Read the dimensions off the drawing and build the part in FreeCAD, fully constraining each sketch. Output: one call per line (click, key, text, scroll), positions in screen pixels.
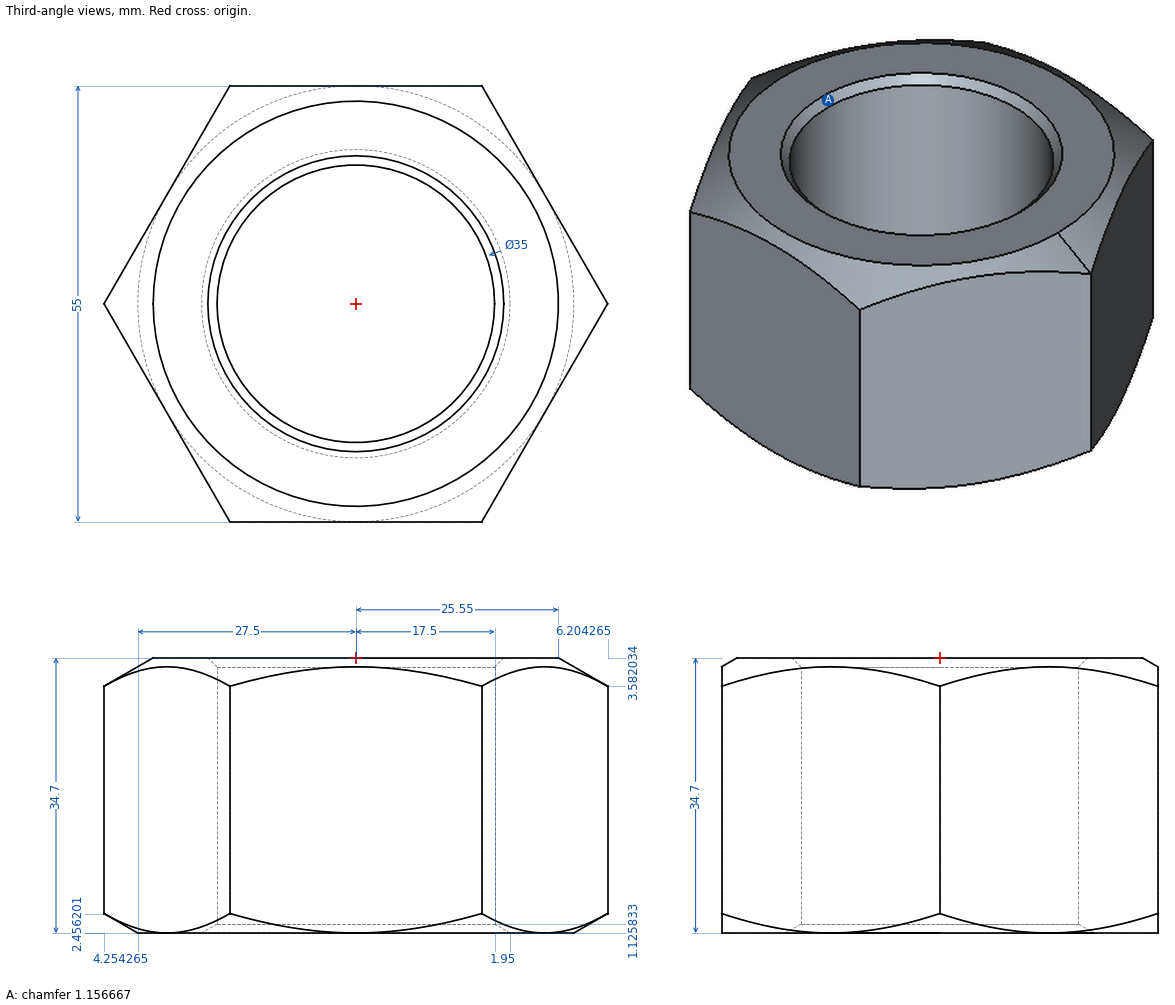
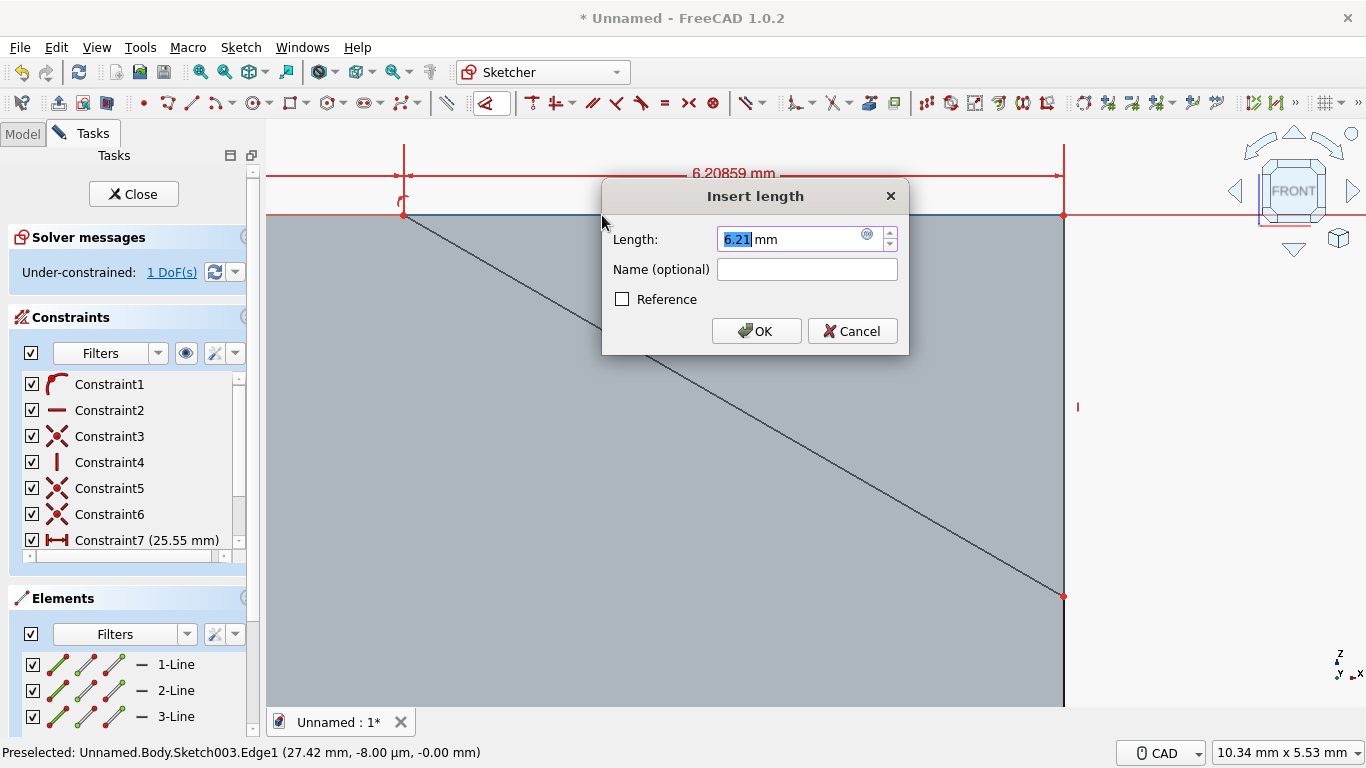
text(6.204265)
key(Return)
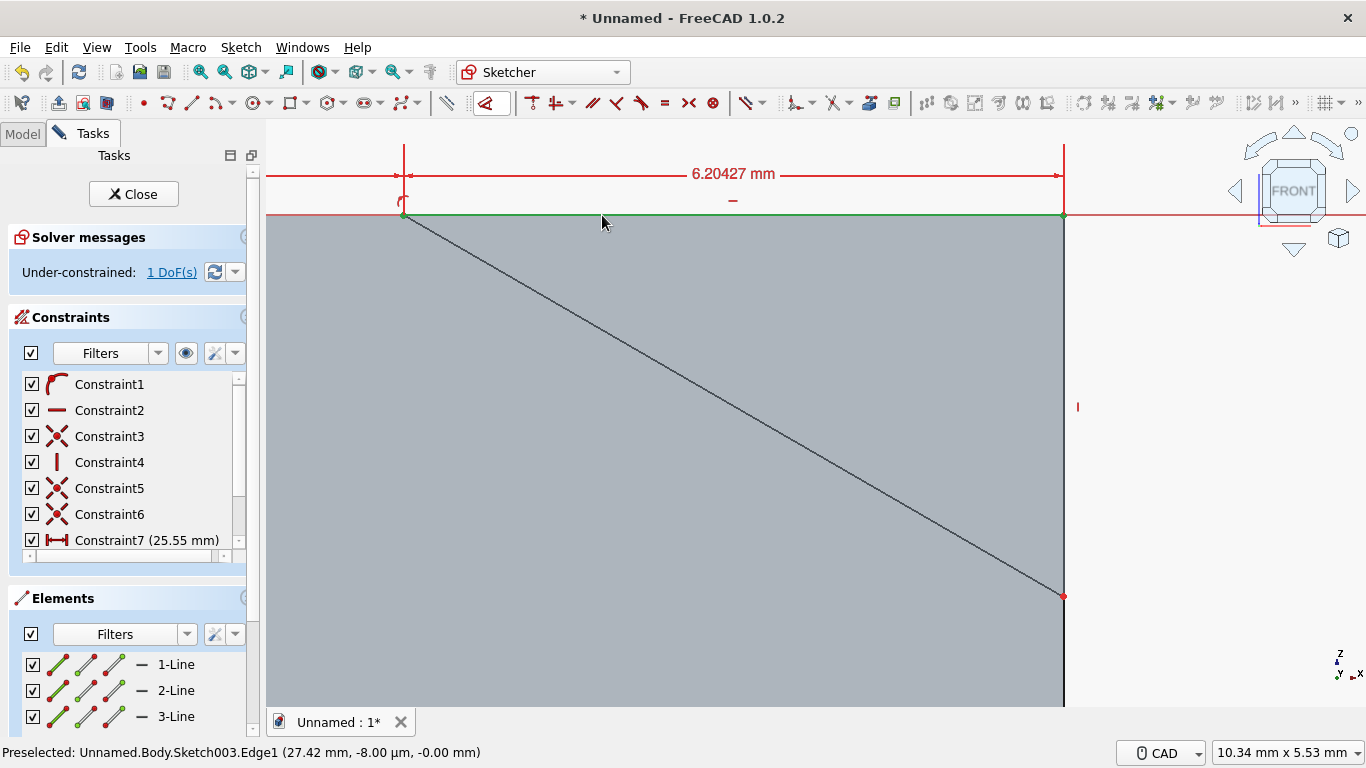
click(1064, 330)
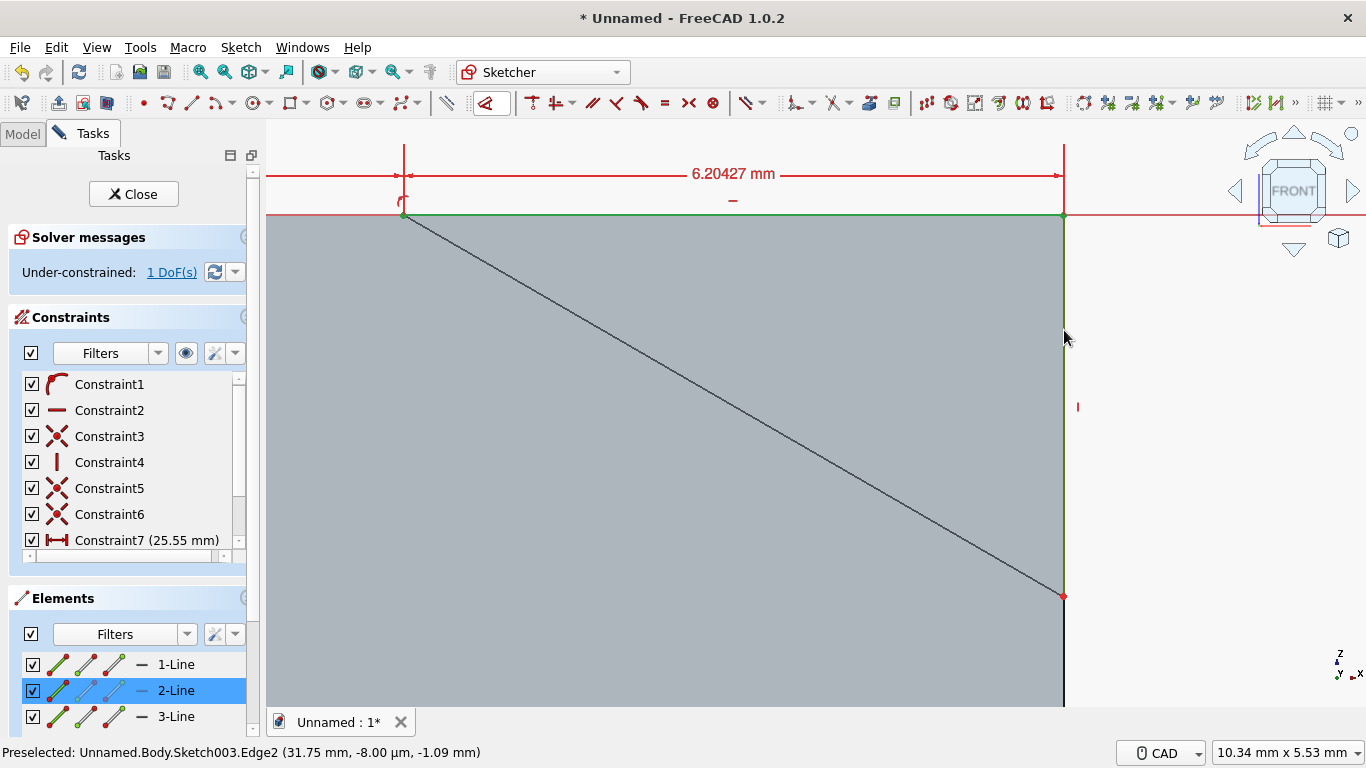
key(i)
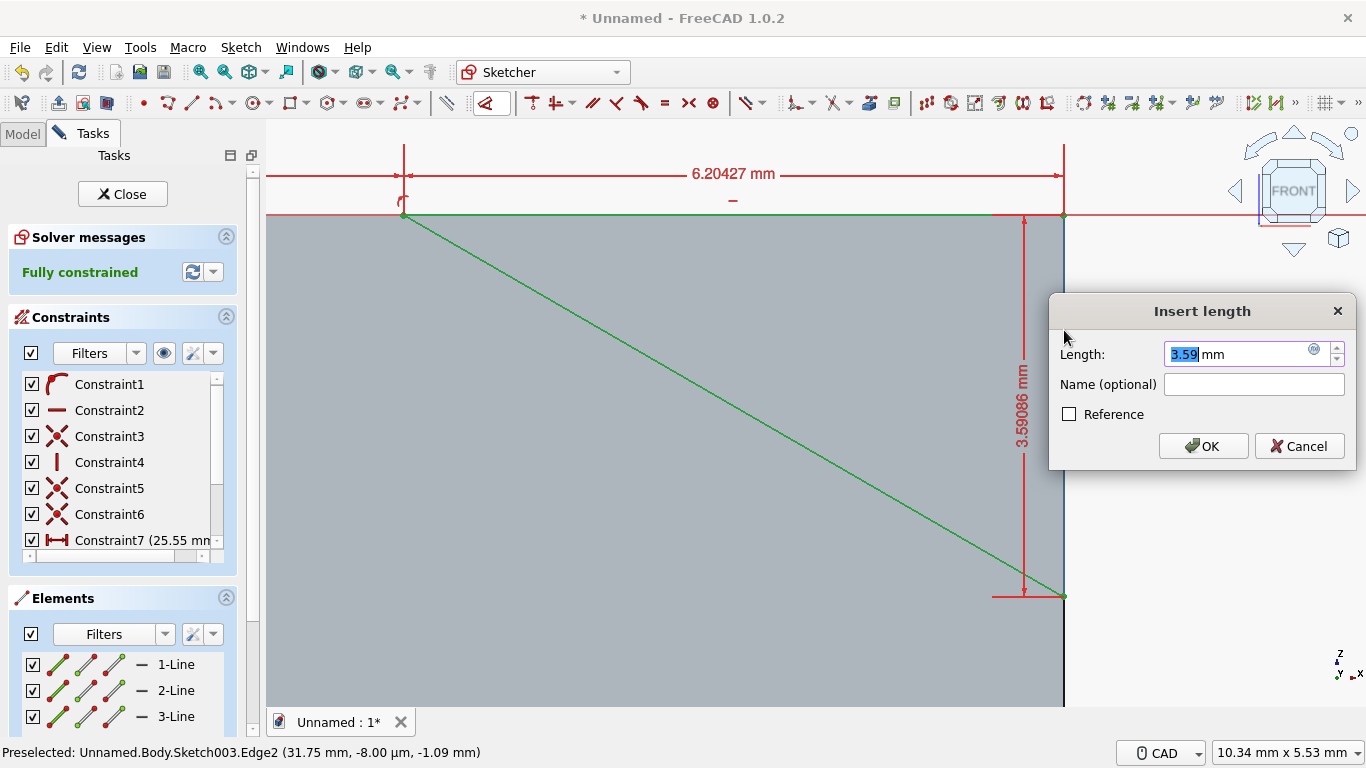
text(3.582034)
key(Return)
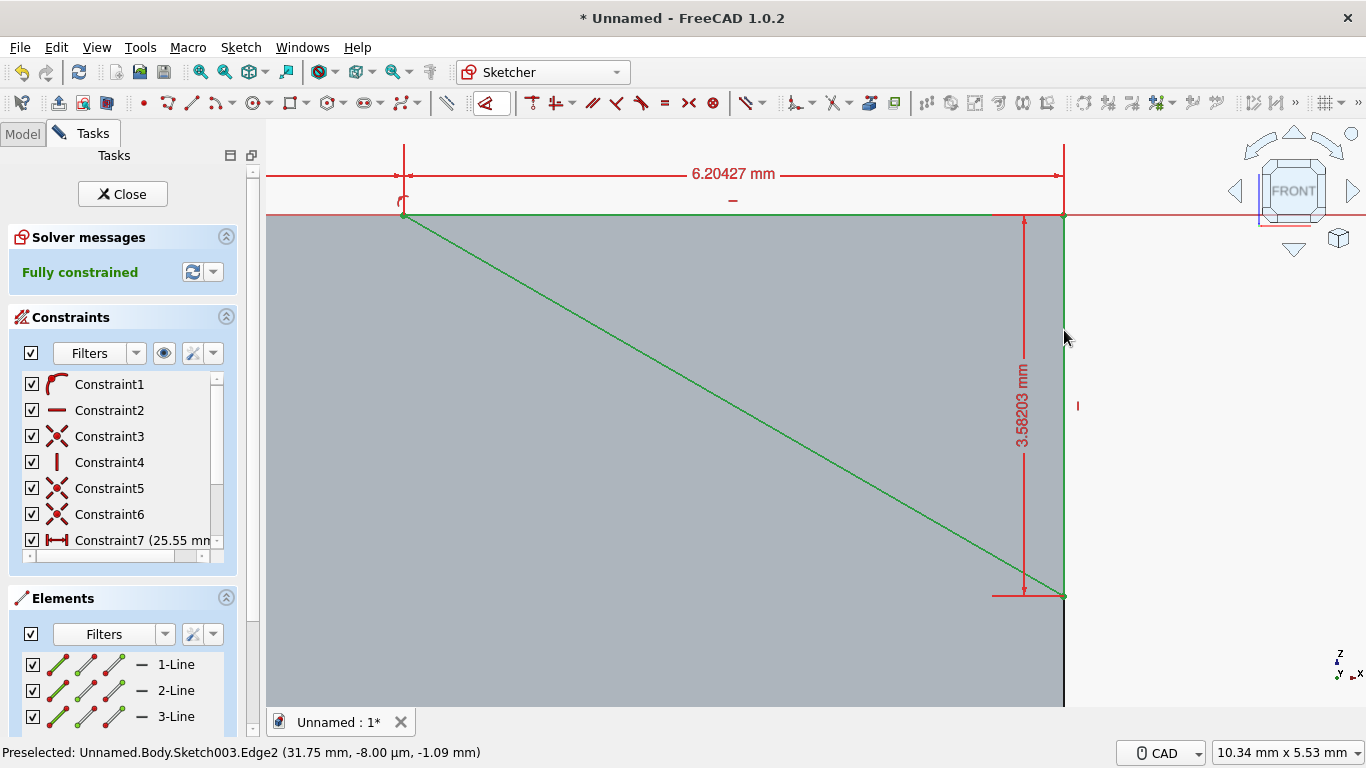
click(123, 194)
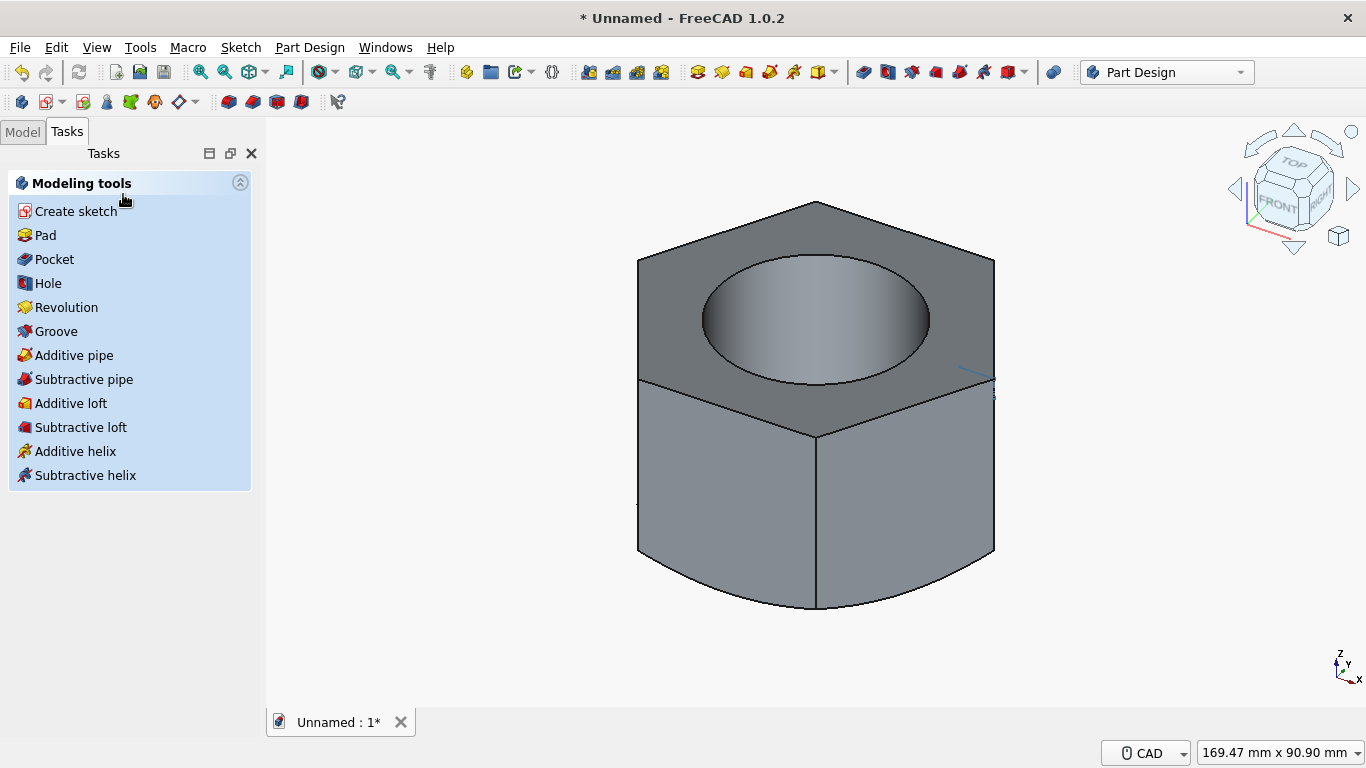
click(912, 72)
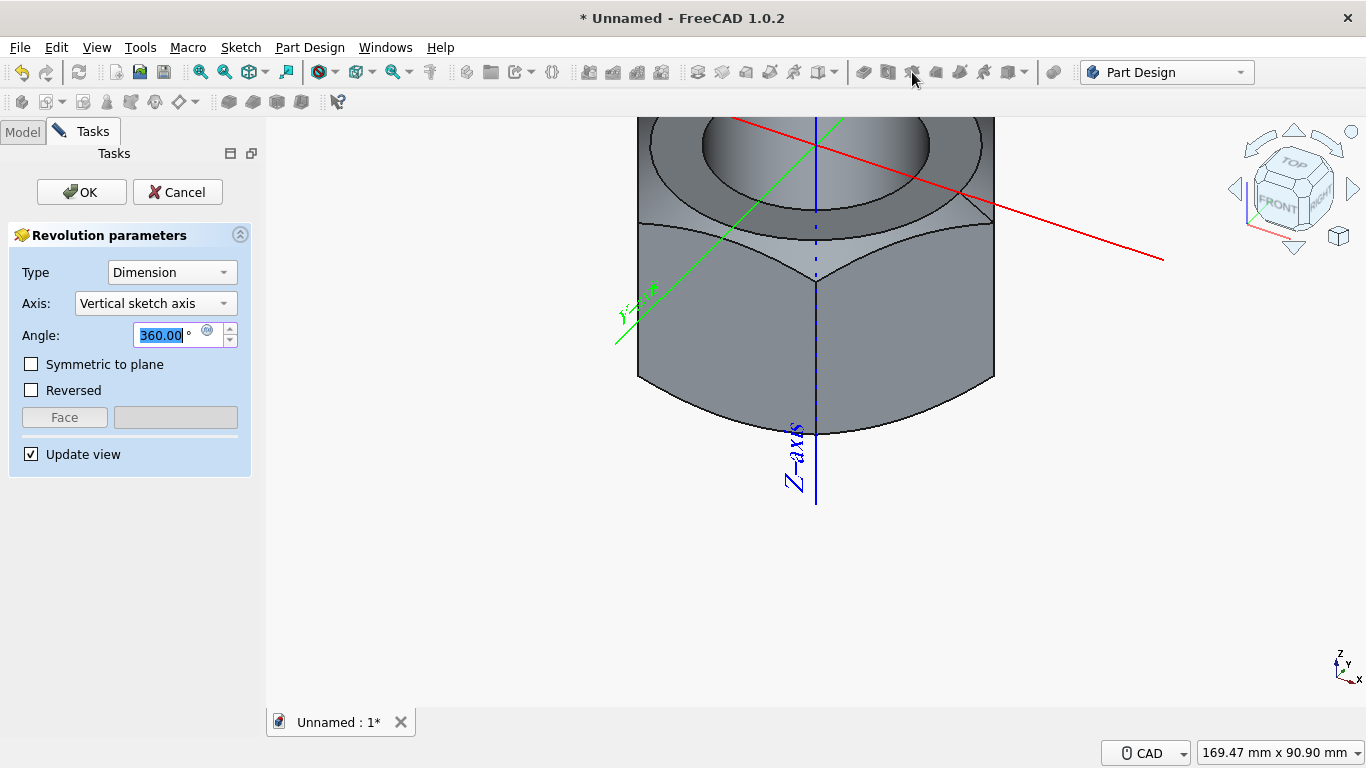
click(82, 192)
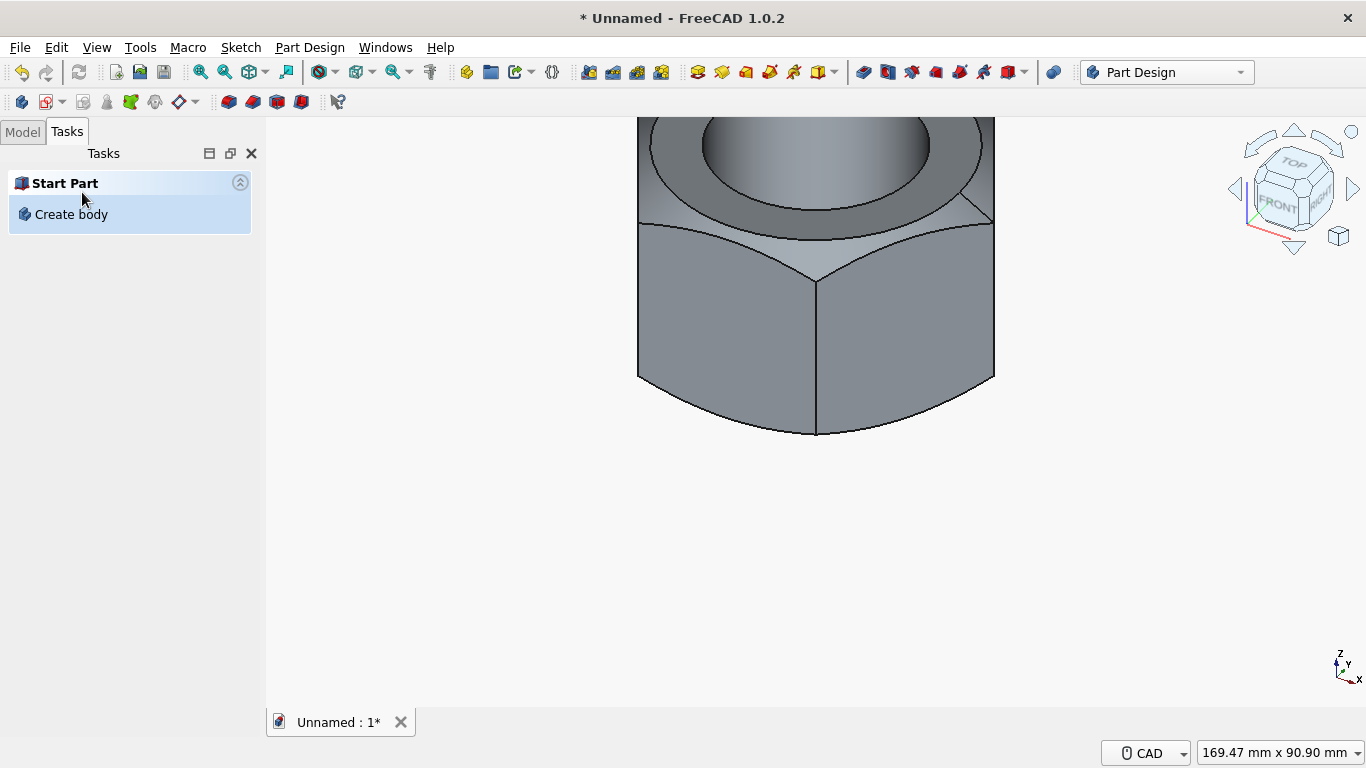
key(v)
key(f)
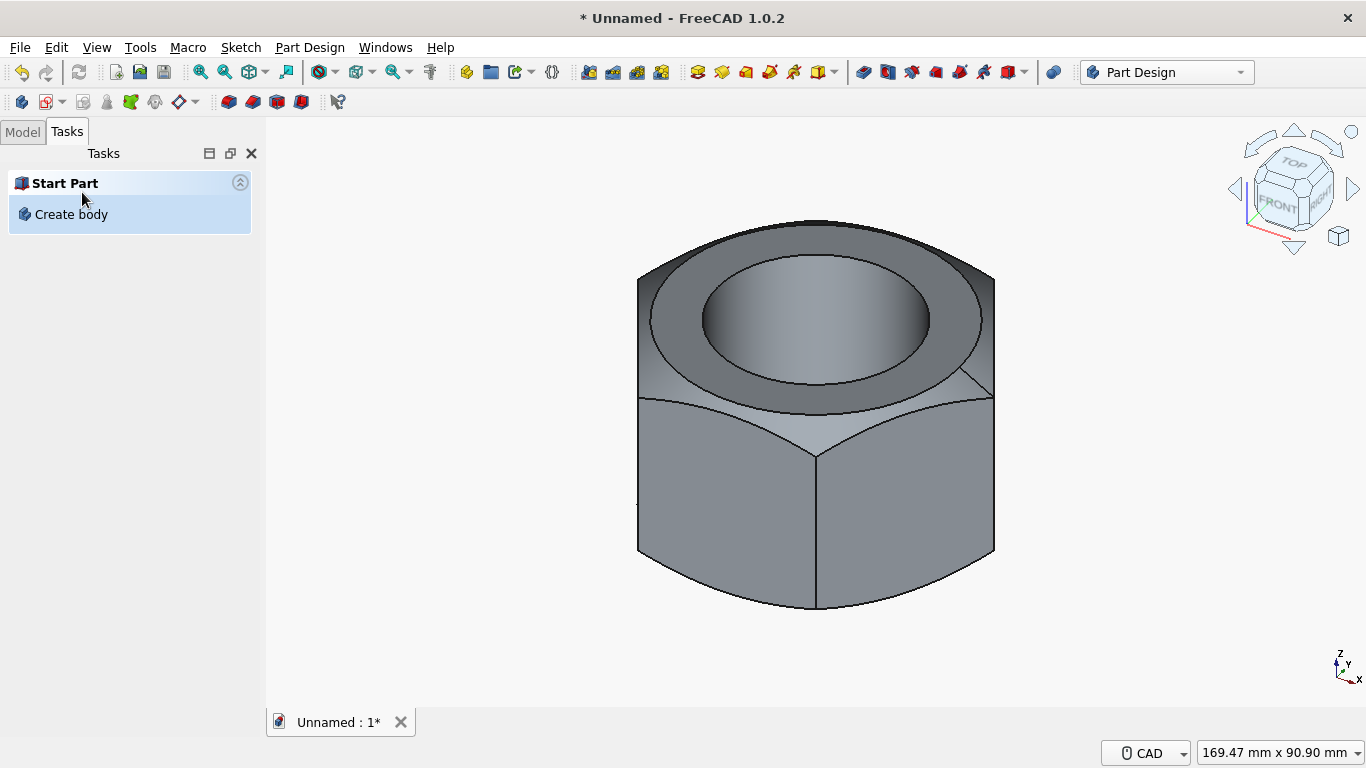
click(718, 286)